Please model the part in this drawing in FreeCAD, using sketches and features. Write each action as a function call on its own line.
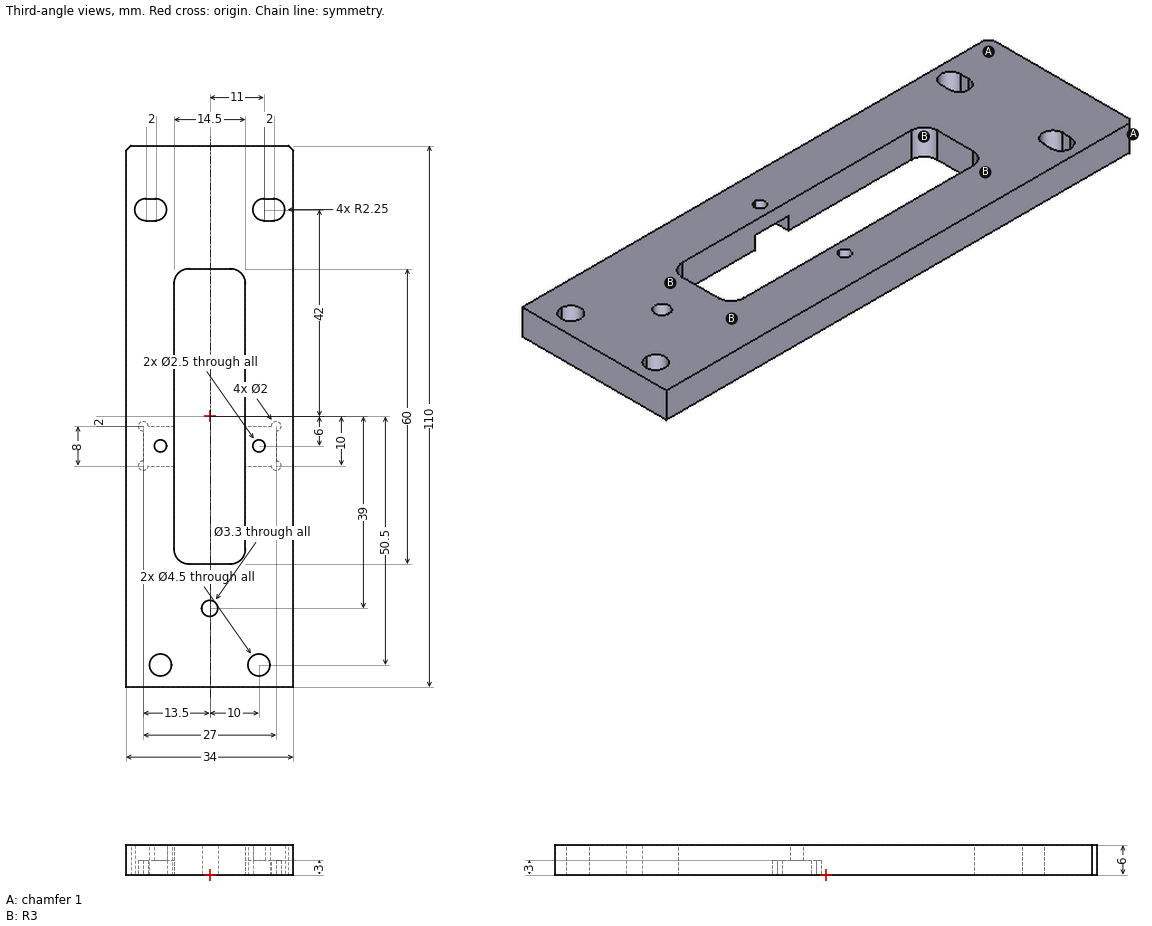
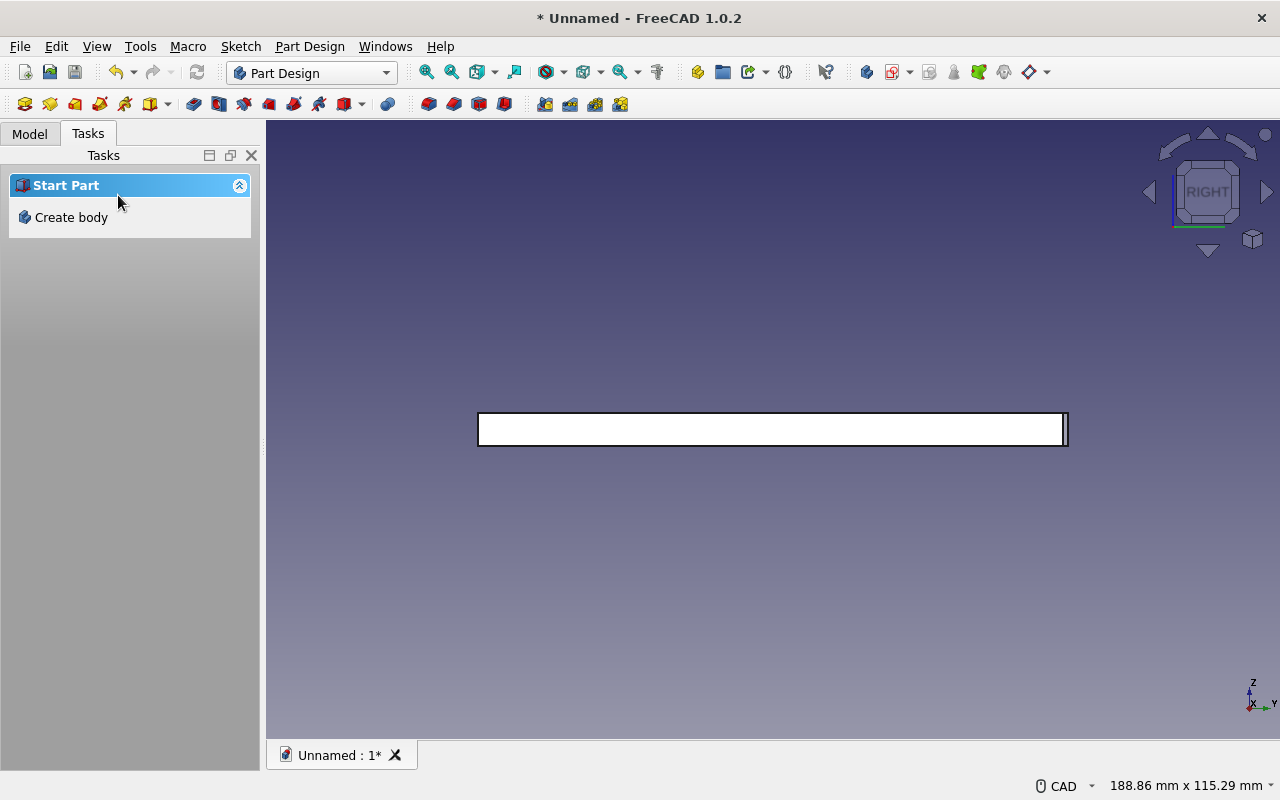
key(5)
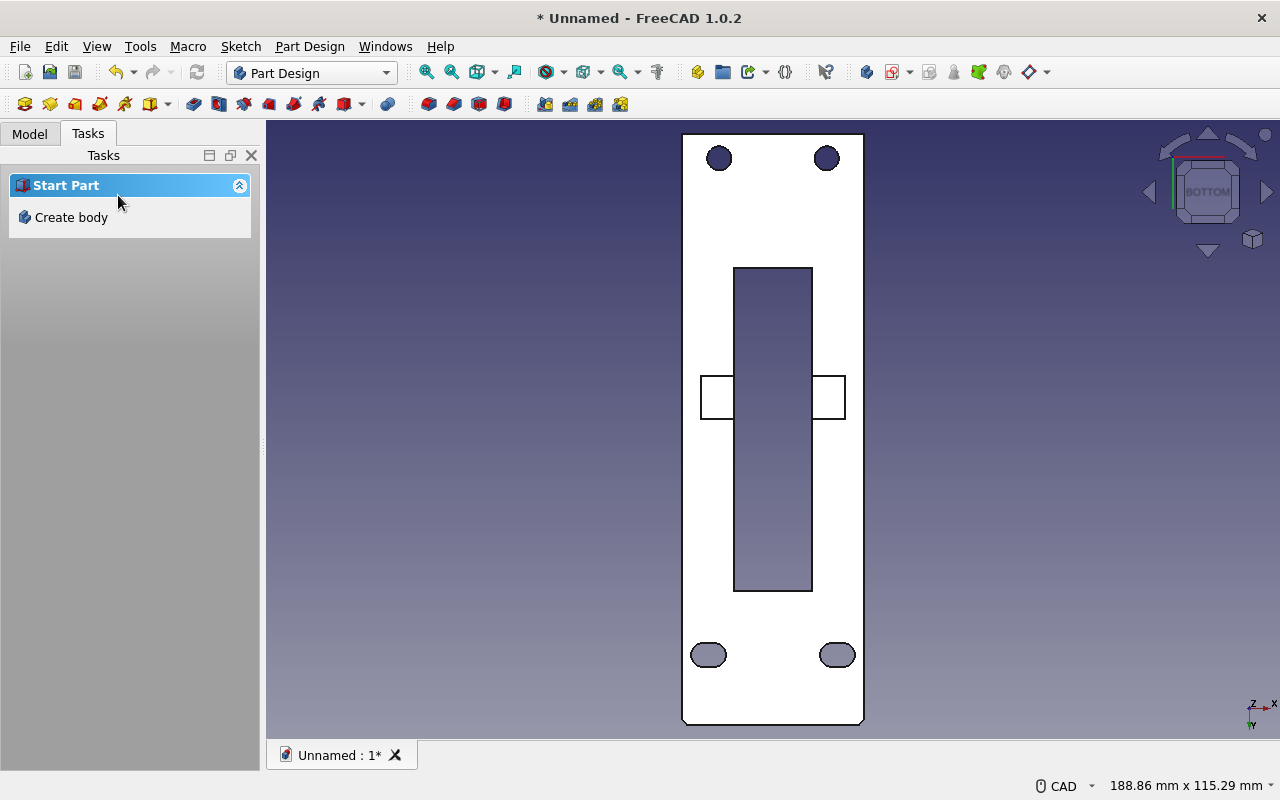
key(4)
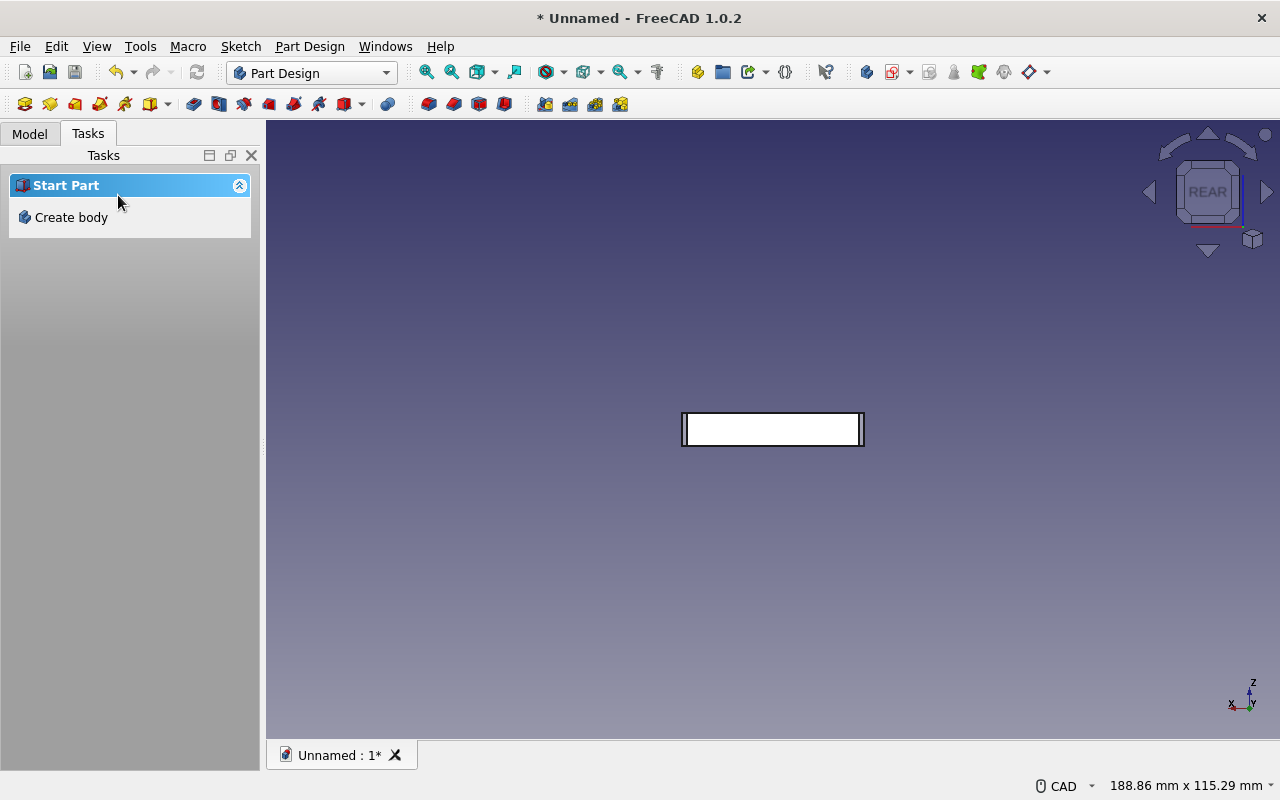
key(v)
key(f)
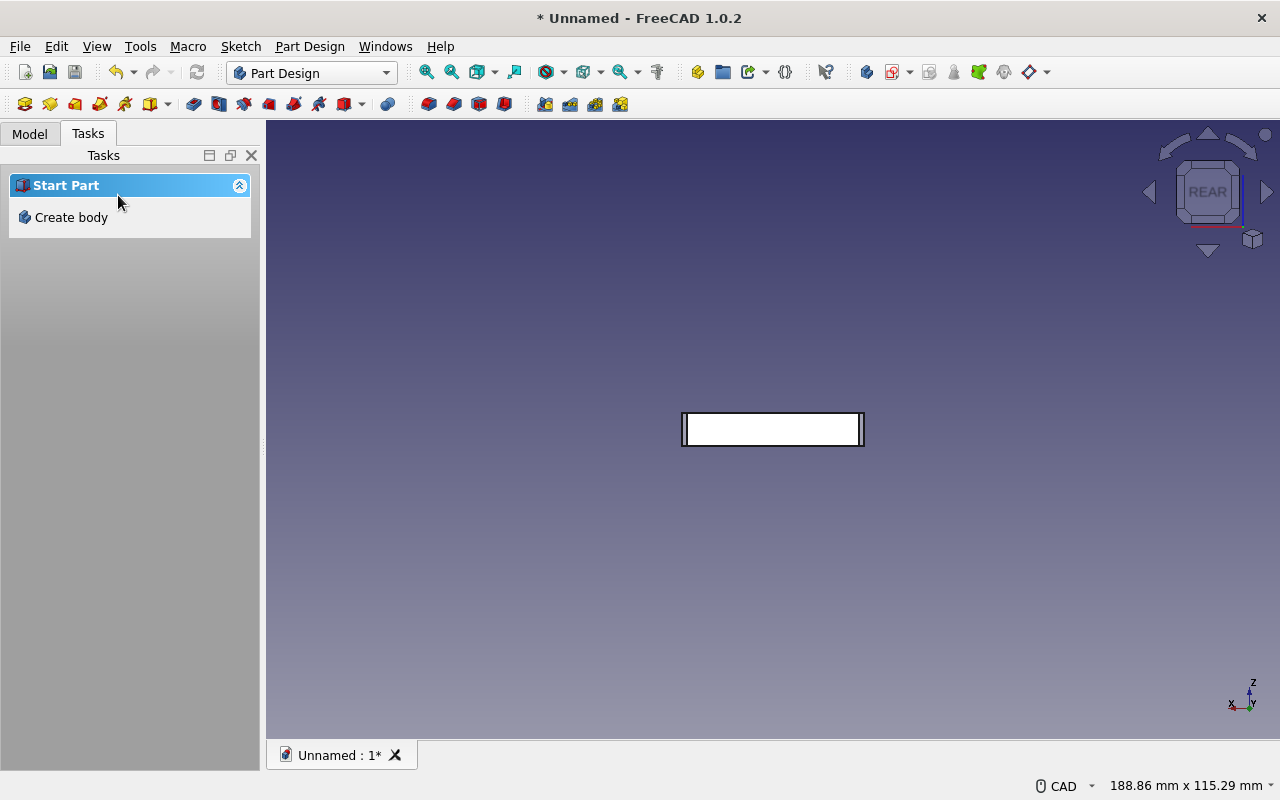
key(6)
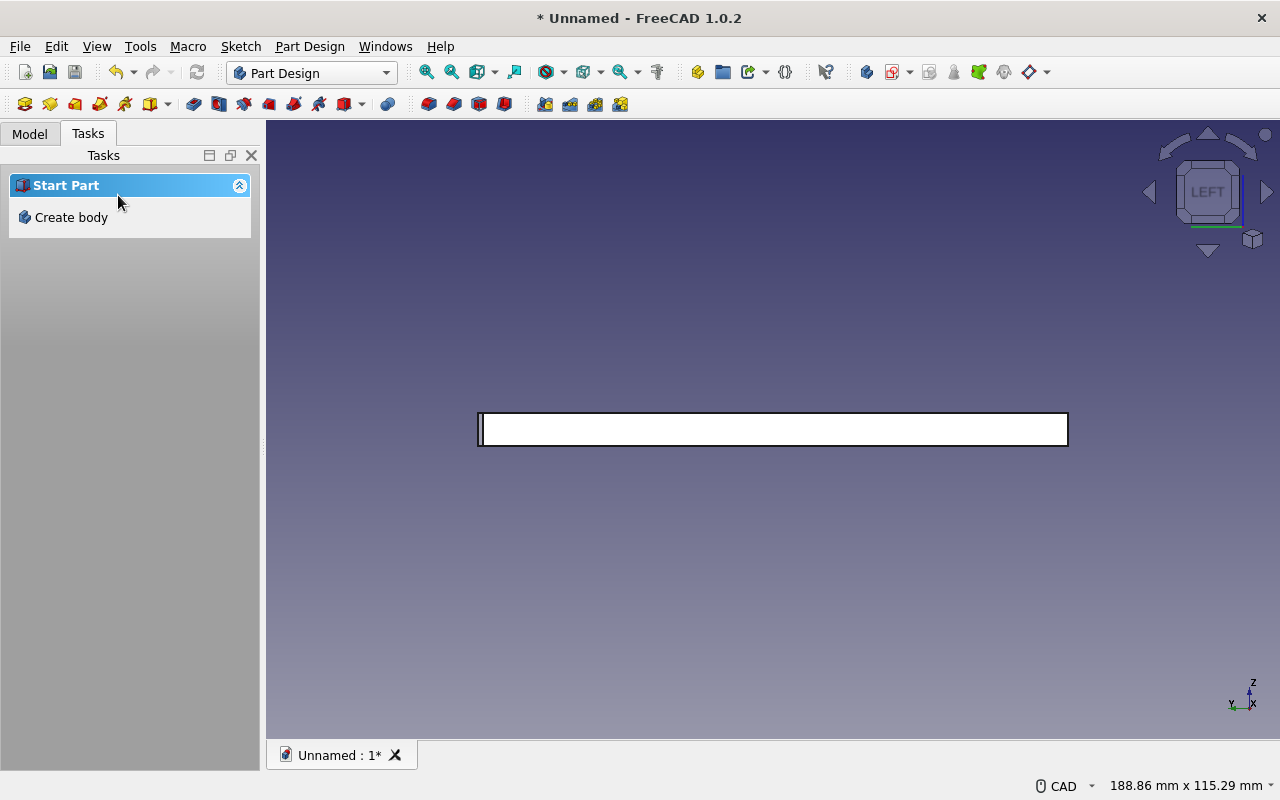
key(v)
key(3)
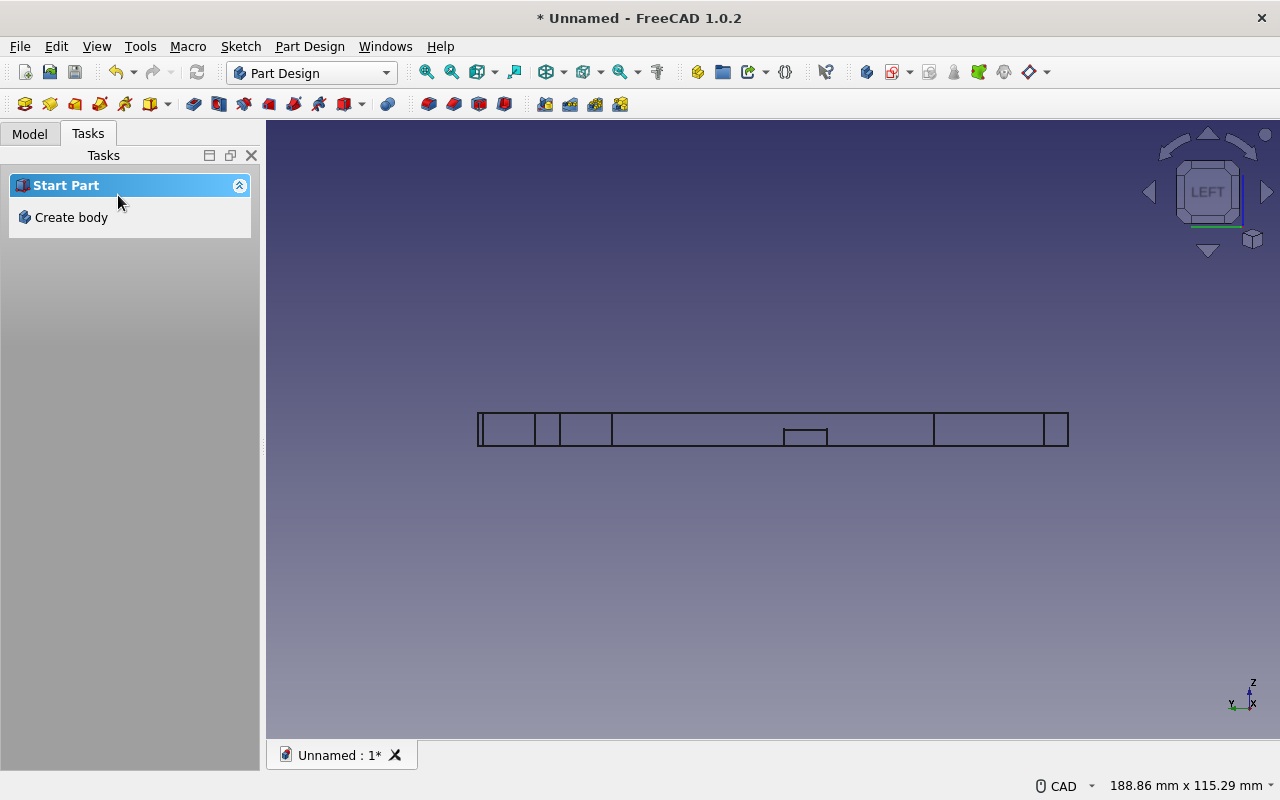
key(0)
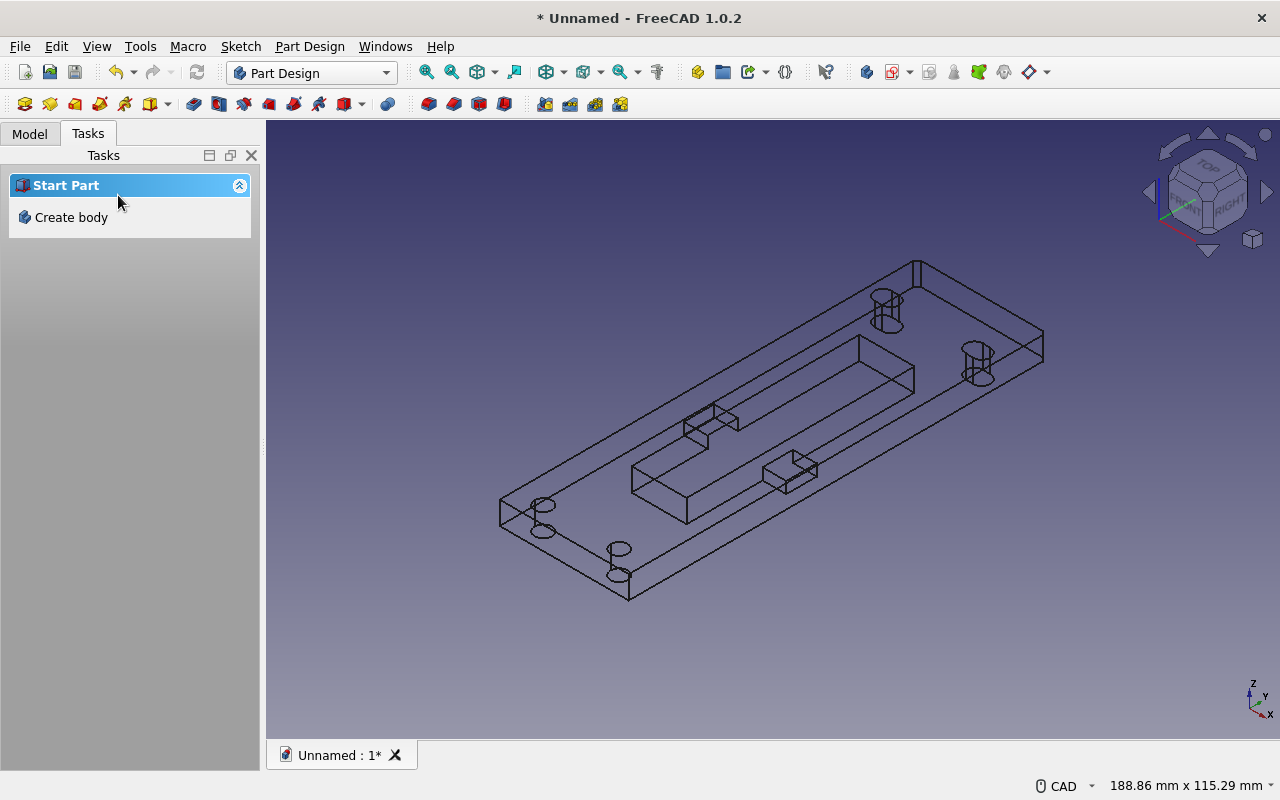
click(859, 347)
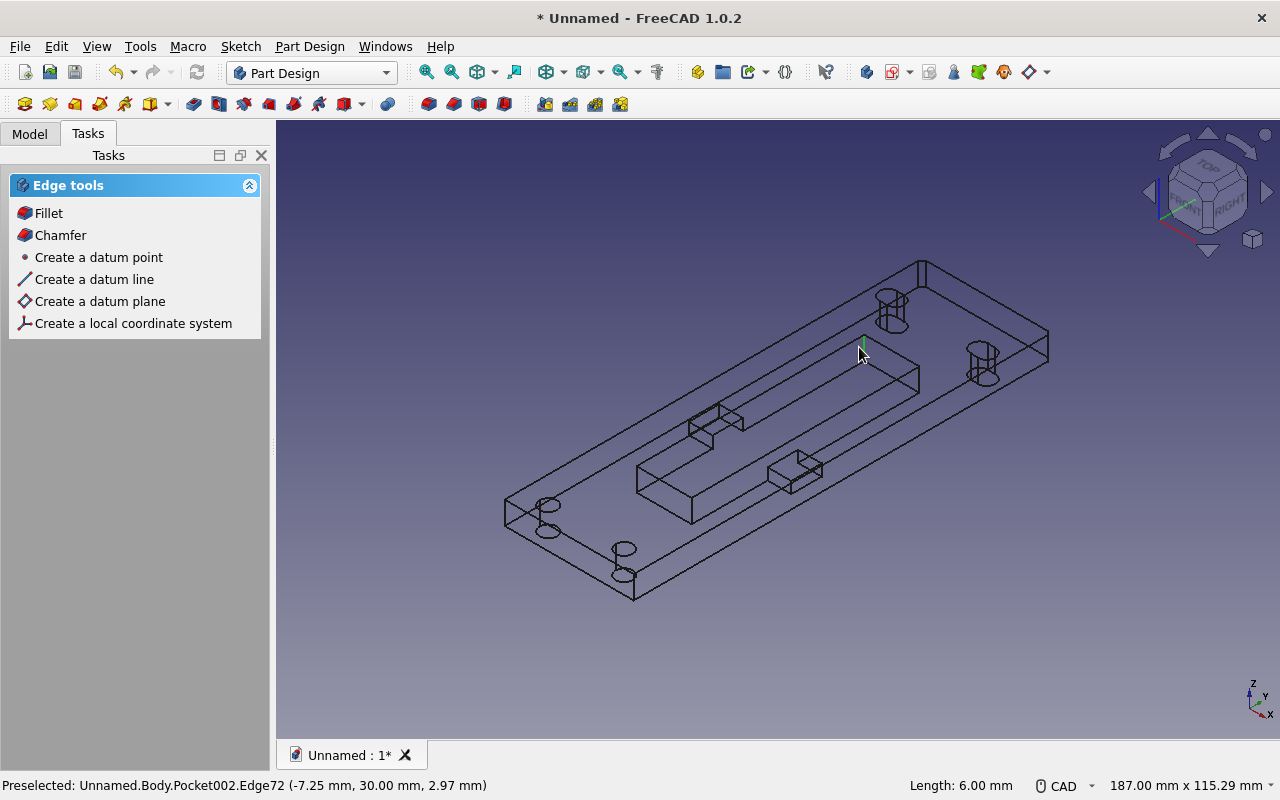
click(637, 478, ctrl)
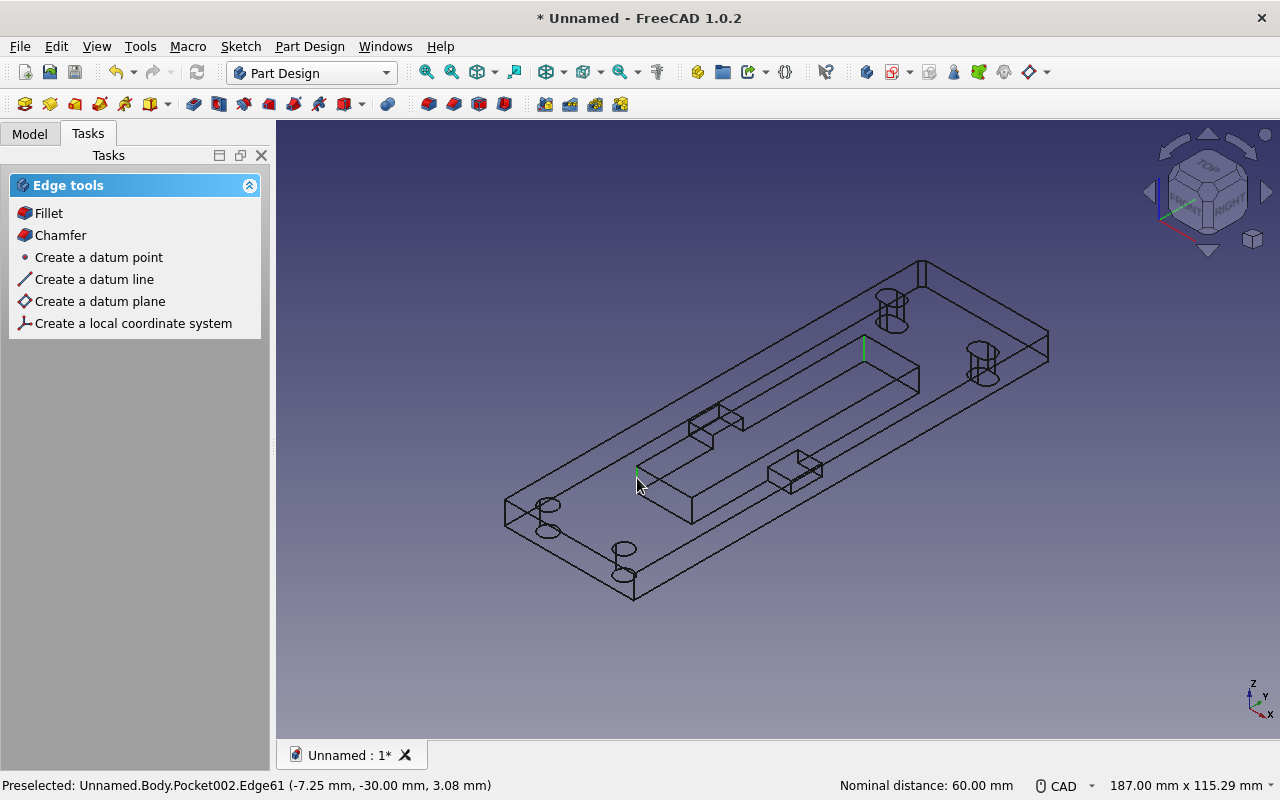
click(692, 510, ctrl)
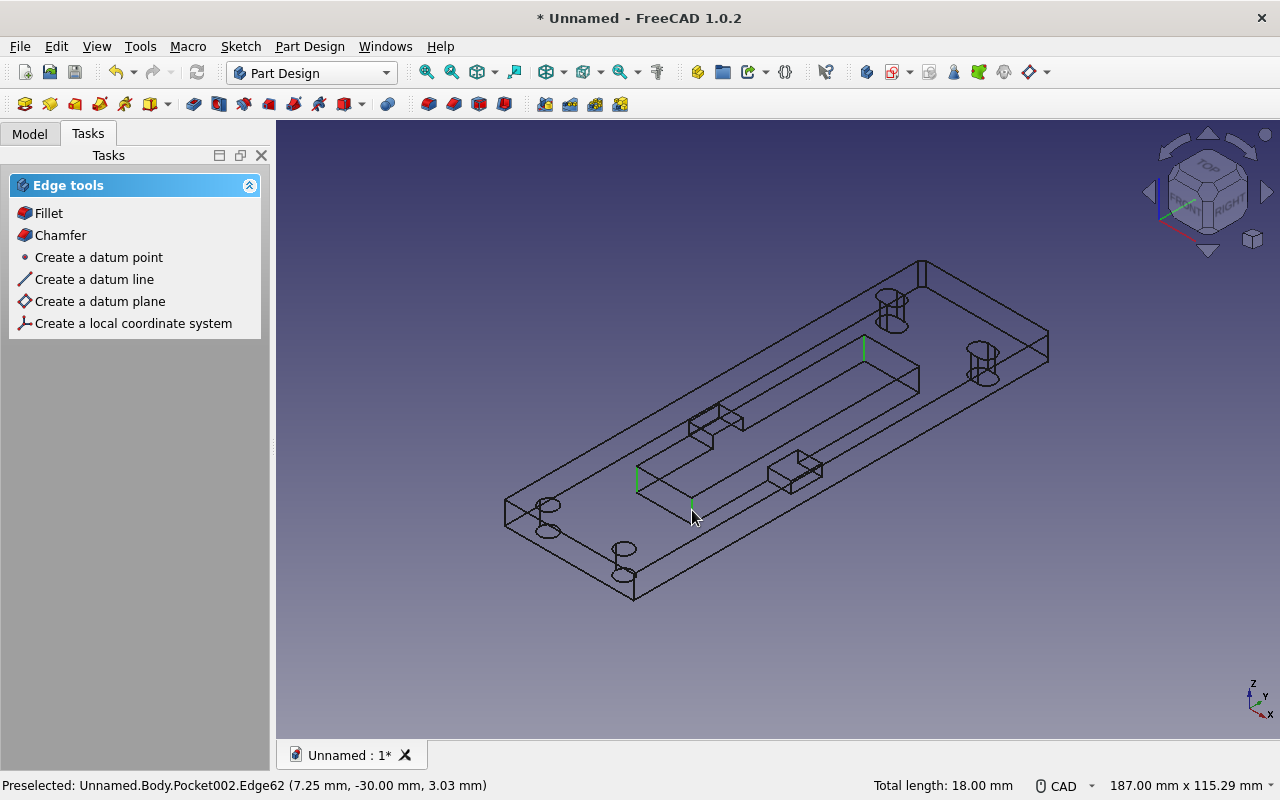
click(919, 379, ctrl)